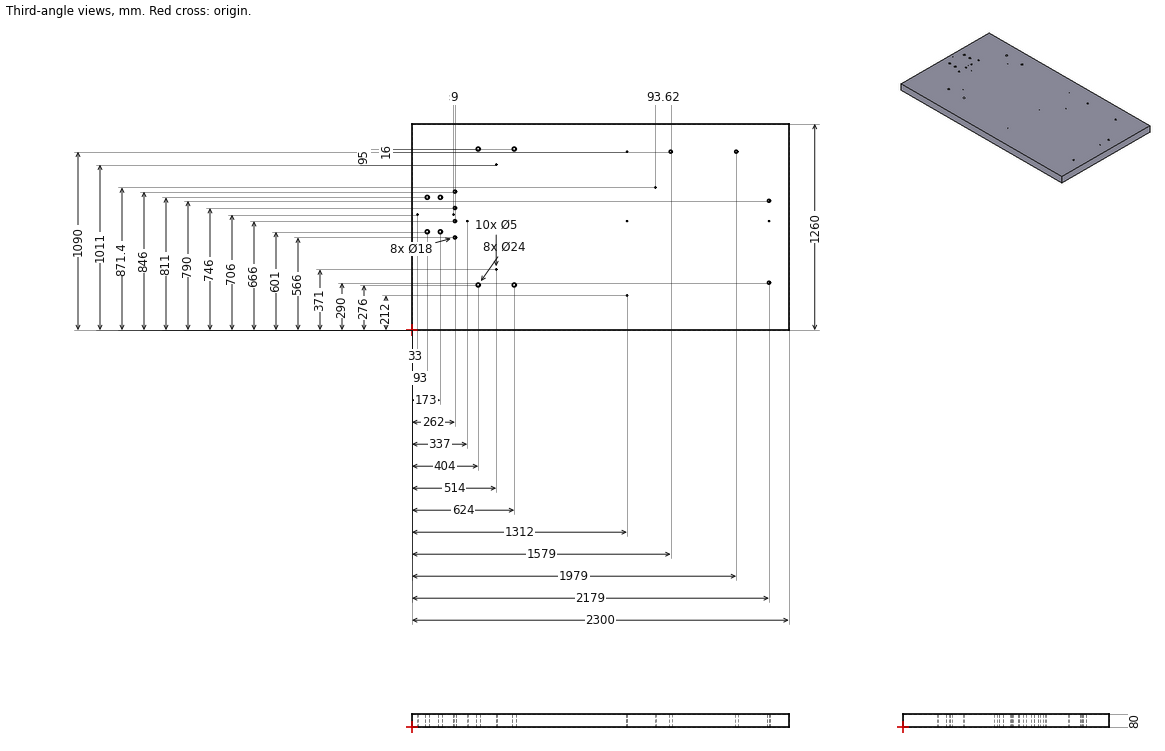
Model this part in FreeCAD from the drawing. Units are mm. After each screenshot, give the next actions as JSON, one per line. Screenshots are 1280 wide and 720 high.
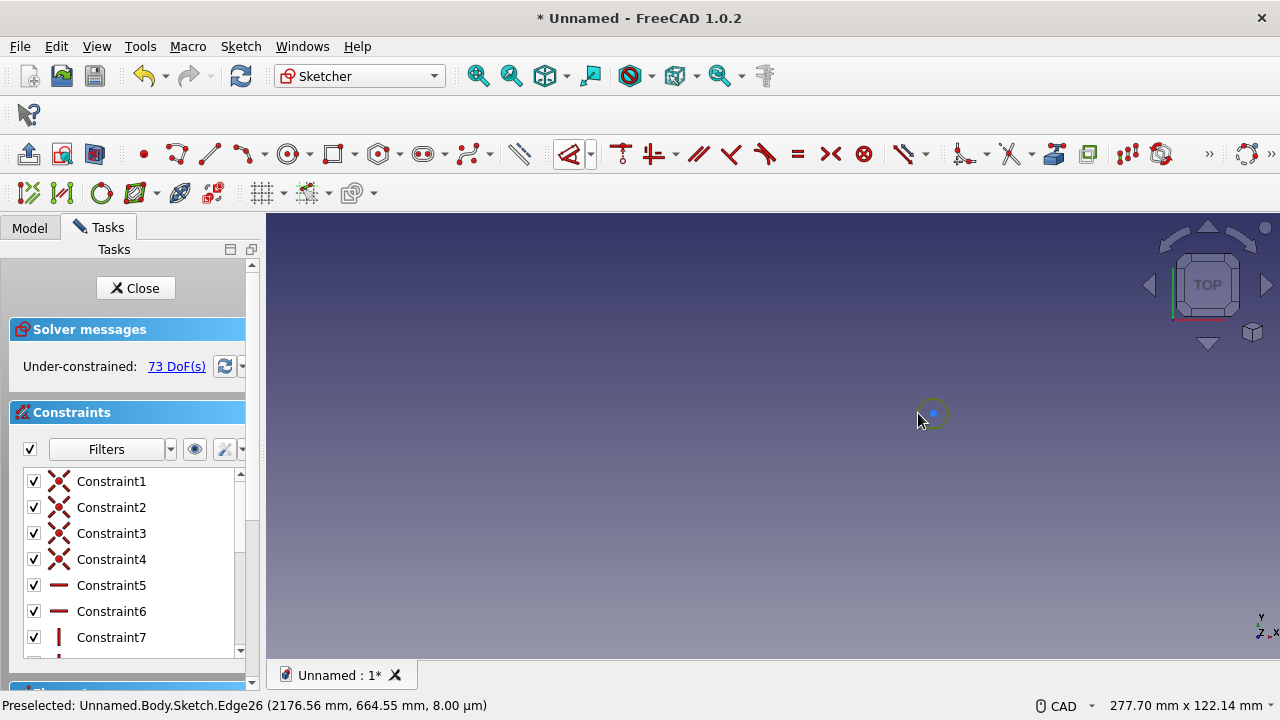
{"action": "scroll", "coordinate": [933, 430], "scroll_direction": "down", "scroll_amount": 14}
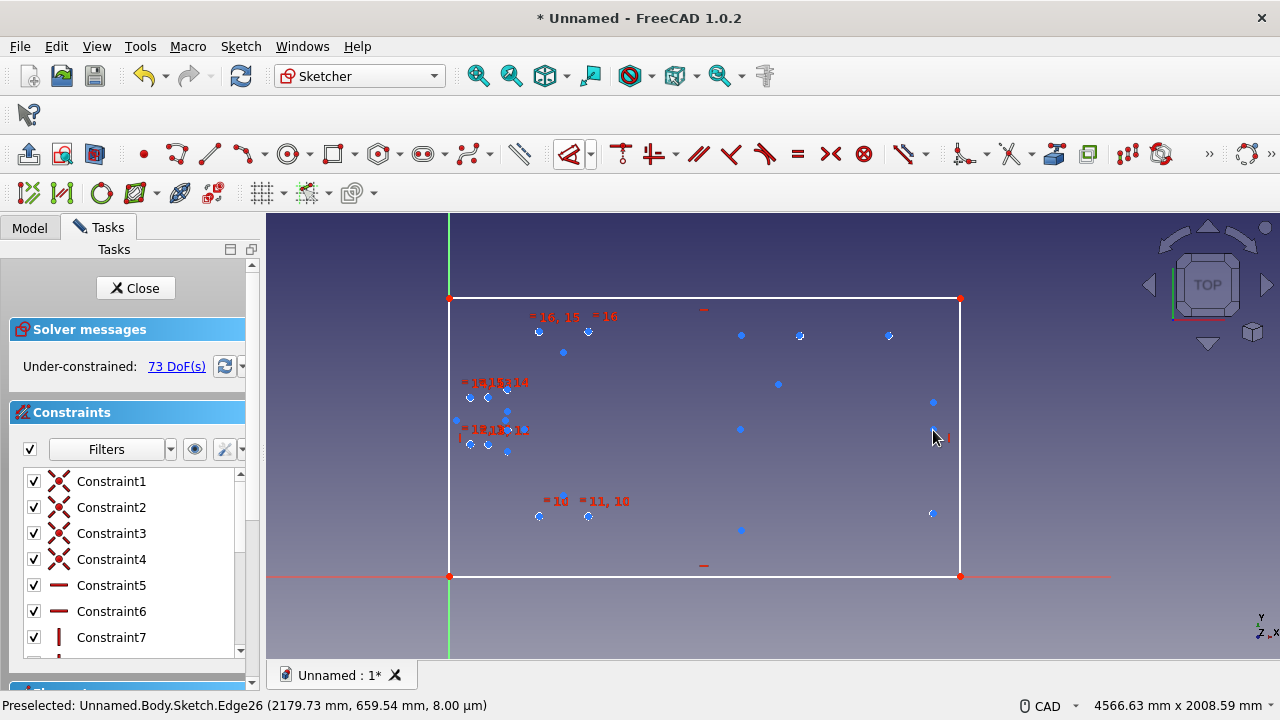
{"action": "scroll", "coordinate": [742, 335], "scroll_direction": "up", "scroll_amount": 11}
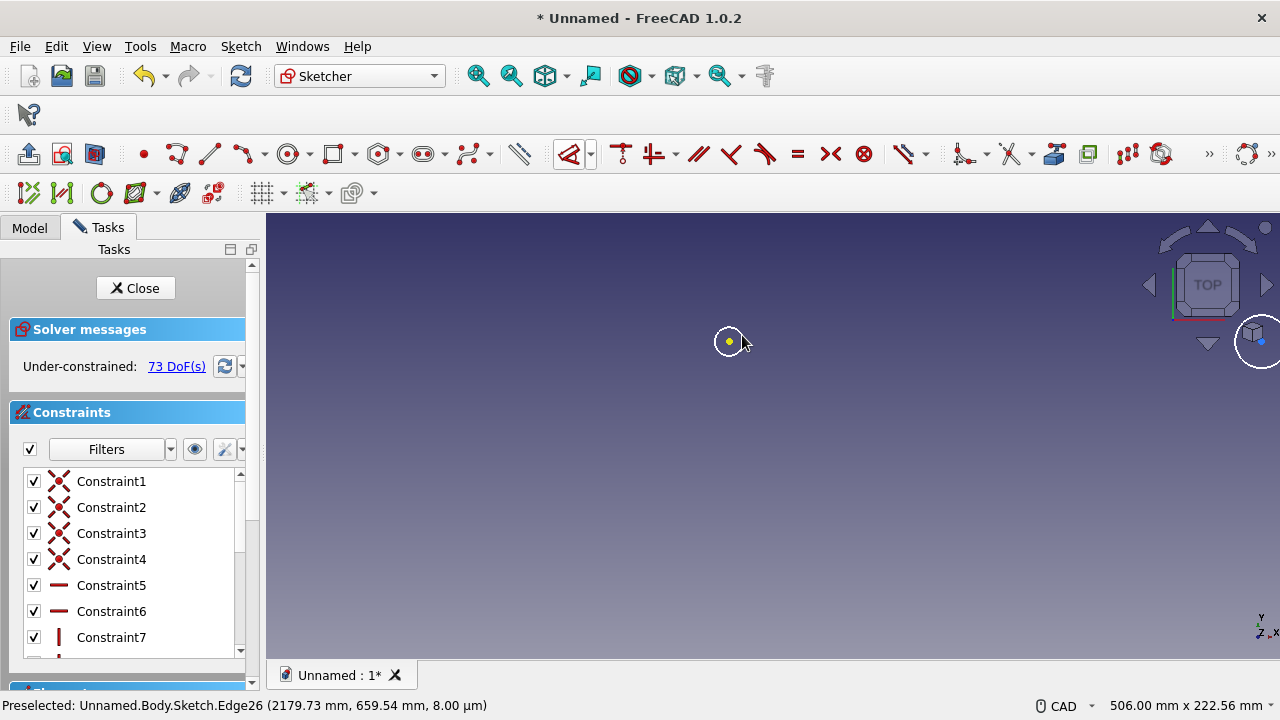
{"action": "left_click", "coordinate": [739, 332]}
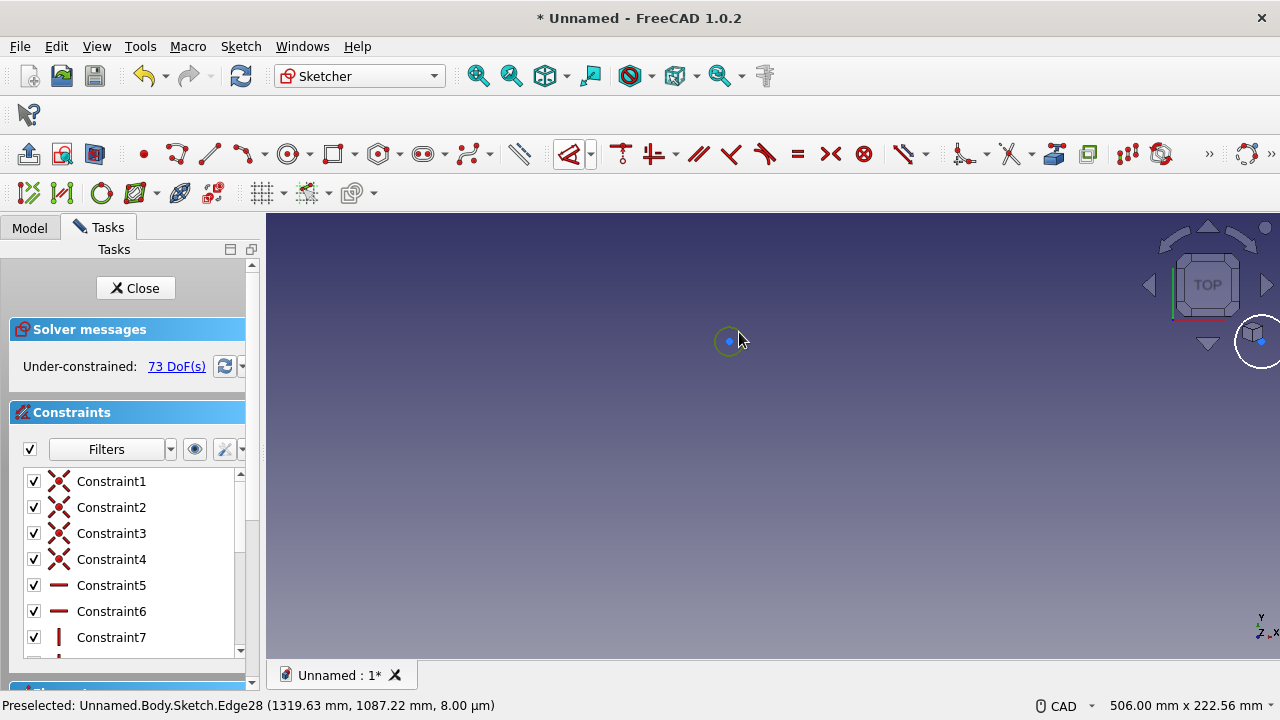
{"action": "left_click", "coordinate": [798, 154]}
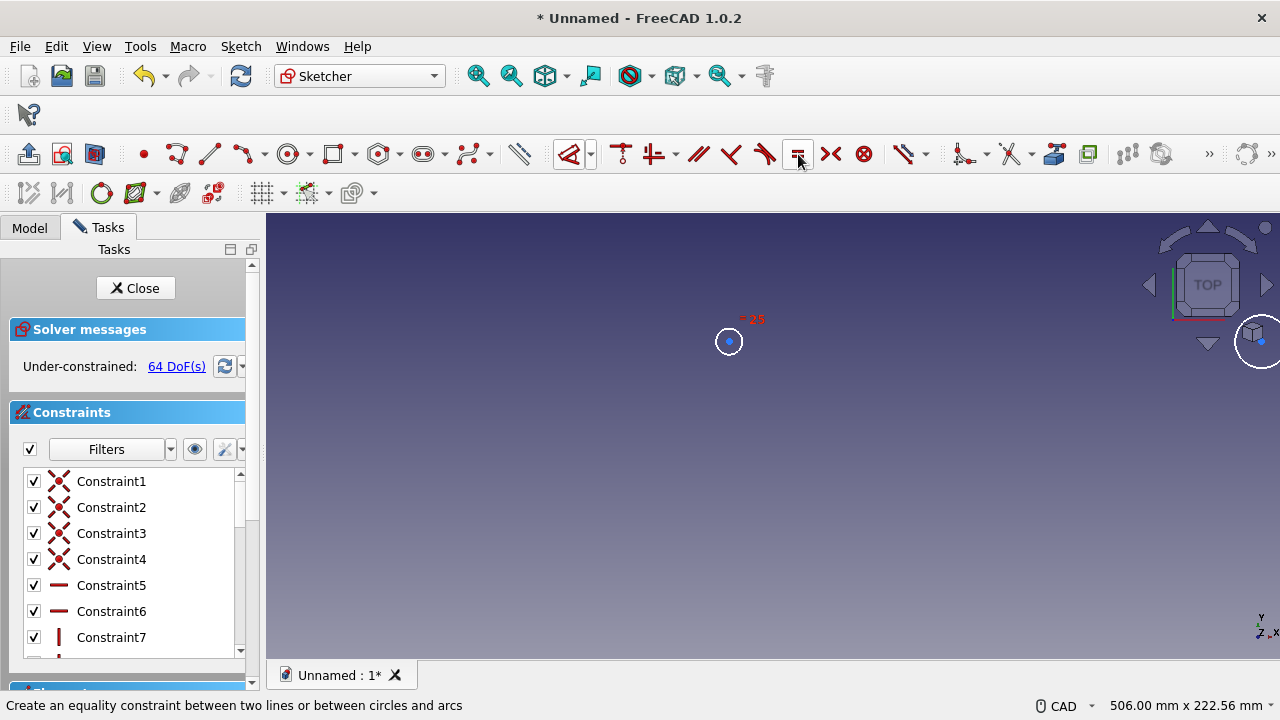
{"action": "scroll", "coordinate": [742, 334], "scroll_direction": "down", "scroll_amount": 11}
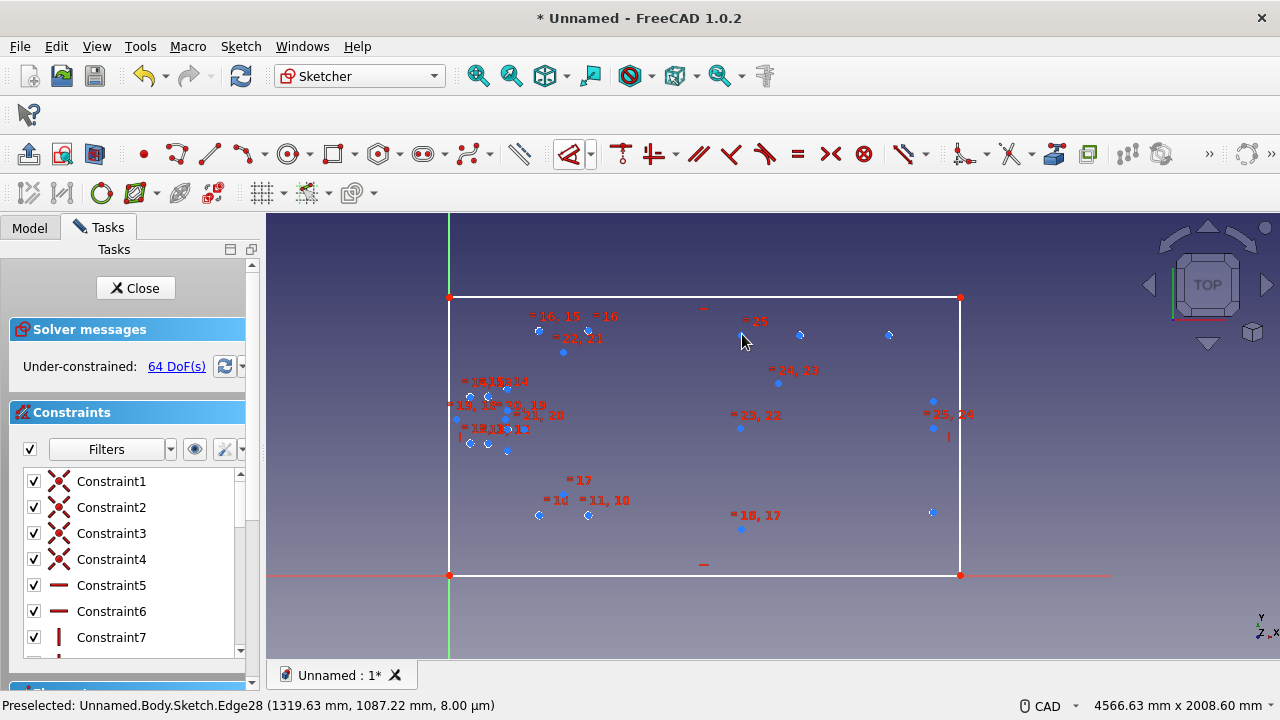
{"action": "scroll", "coordinate": [509, 449], "scroll_direction": "up", "scroll_amount": 9}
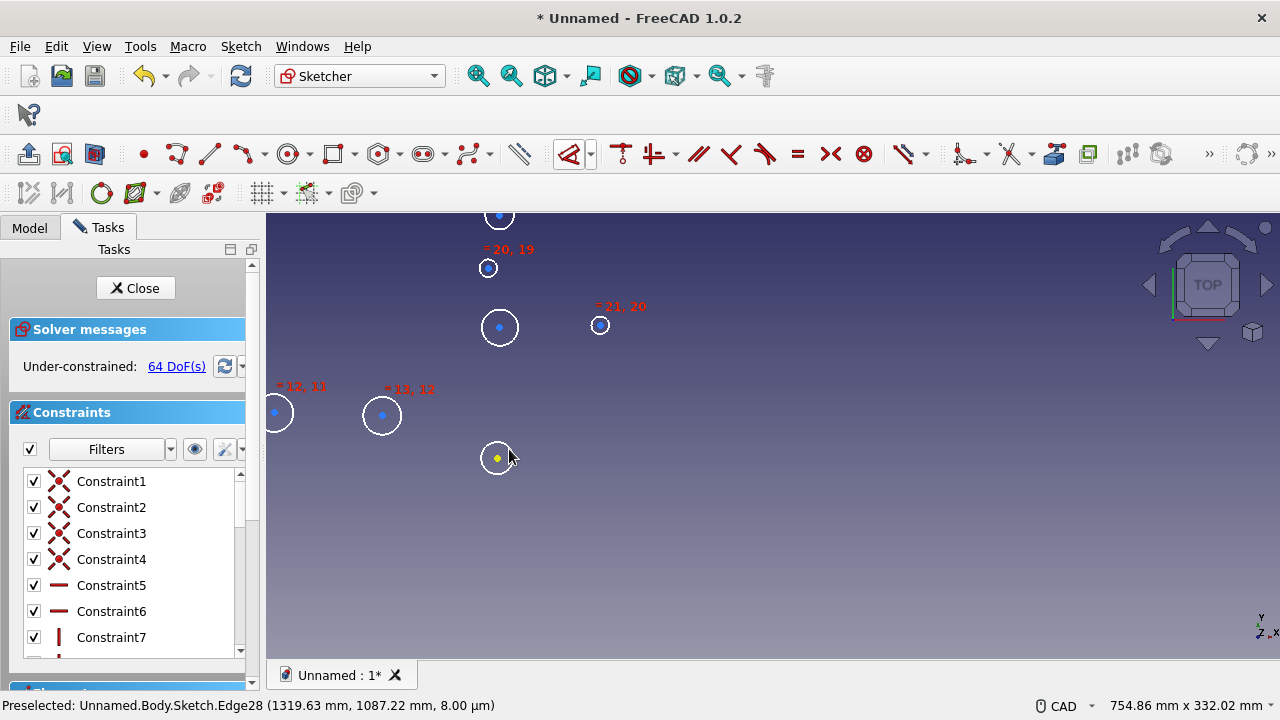
{"action": "left_click", "coordinate": [509, 447]}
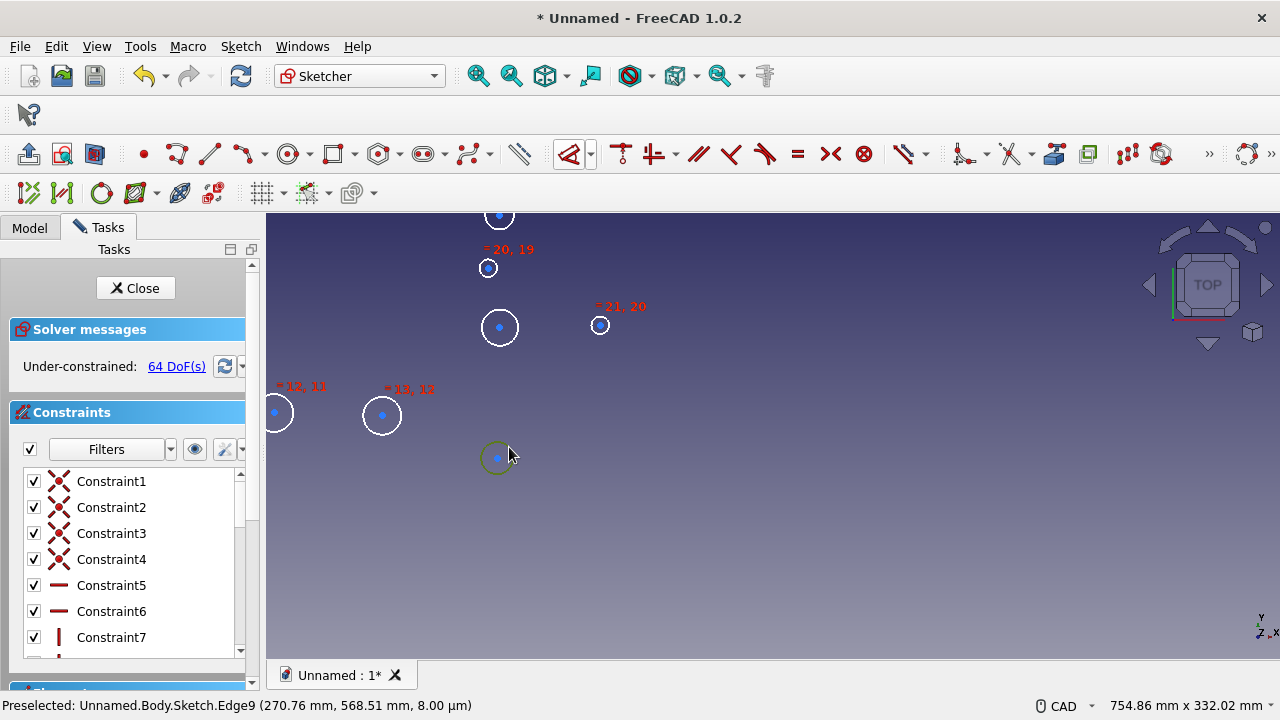
{"action": "scroll", "coordinate": [509, 449], "scroll_direction": "down", "scroll_amount": 9}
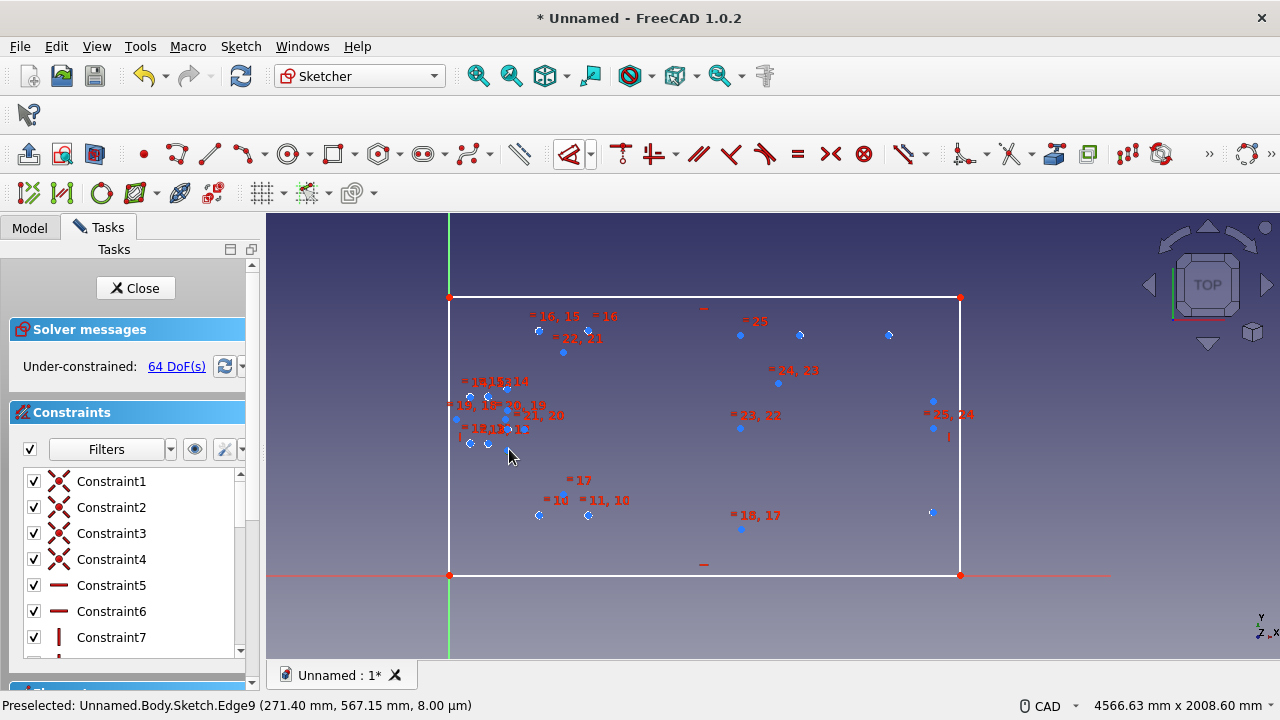
{"action": "scroll", "coordinate": [935, 510], "scroll_direction": "up", "scroll_amount": 8}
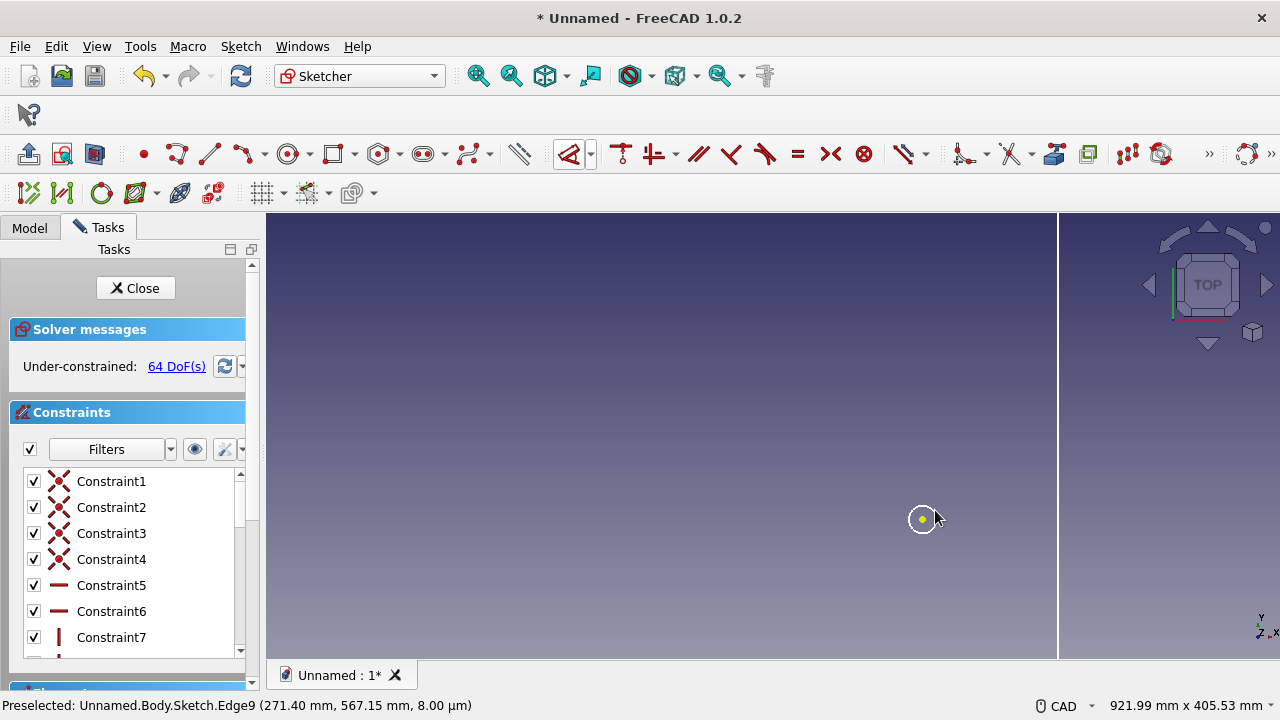
{"action": "left_click", "coordinate": [933, 510]}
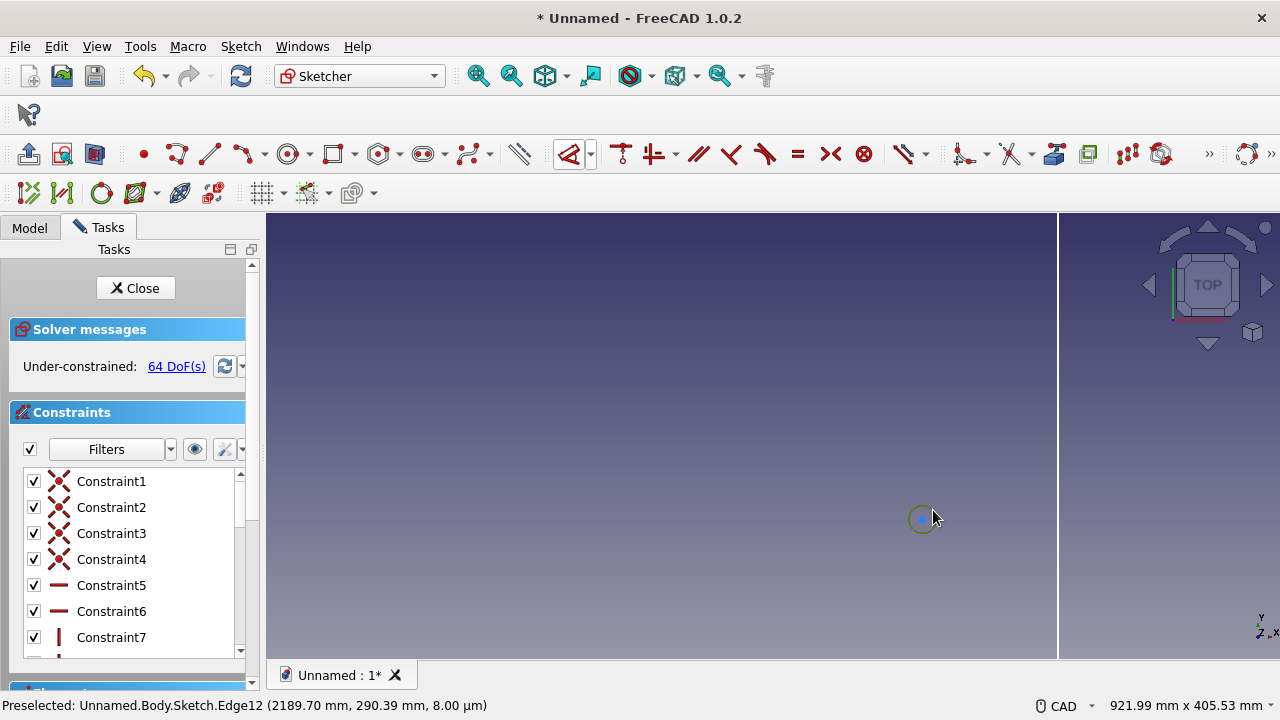
{"action": "scroll", "coordinate": [935, 511], "scroll_direction": "down", "scroll_amount": 8}